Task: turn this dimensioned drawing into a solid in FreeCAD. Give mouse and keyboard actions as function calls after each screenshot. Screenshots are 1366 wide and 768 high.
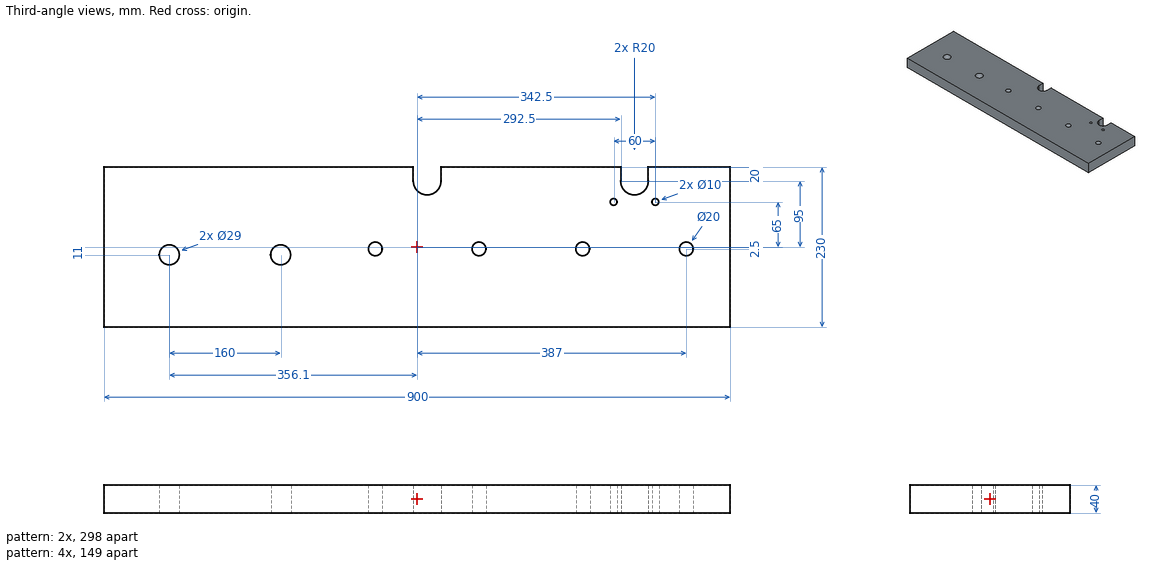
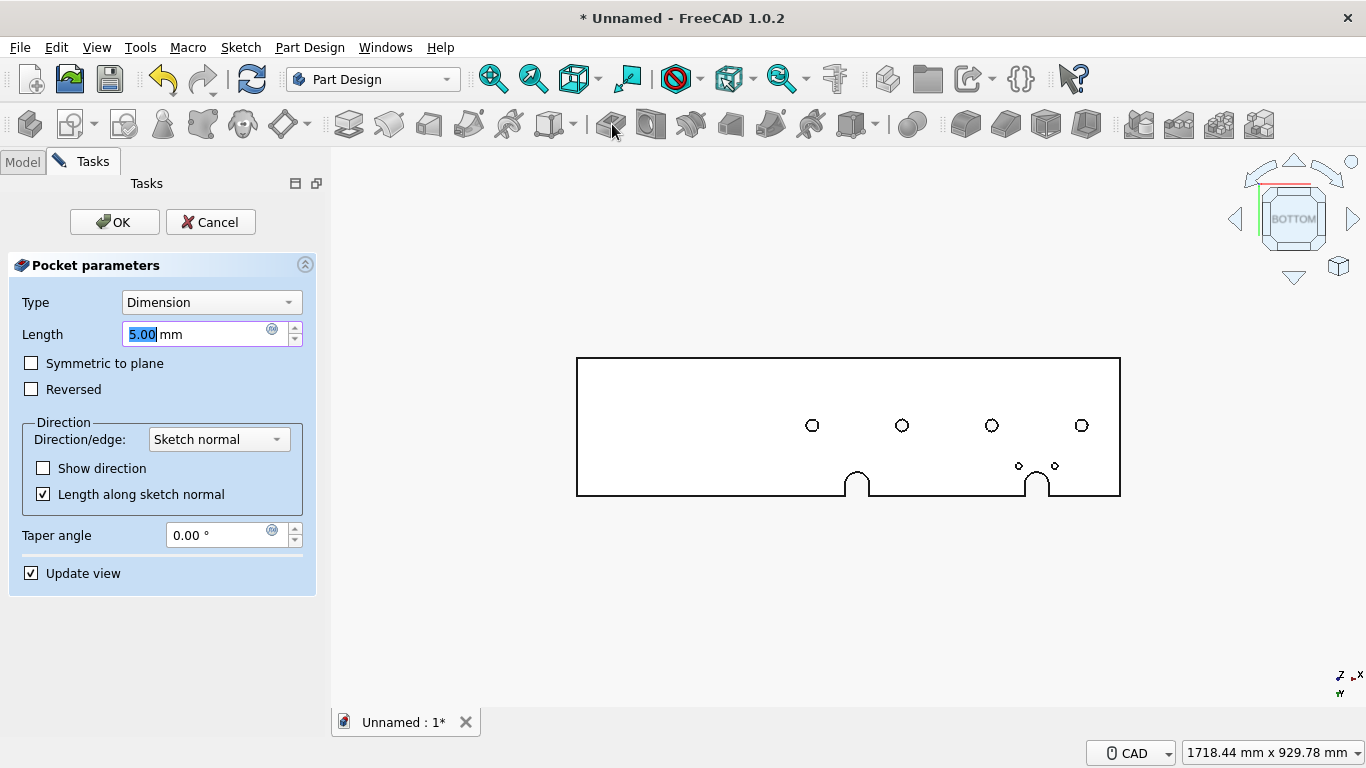
click(212, 302)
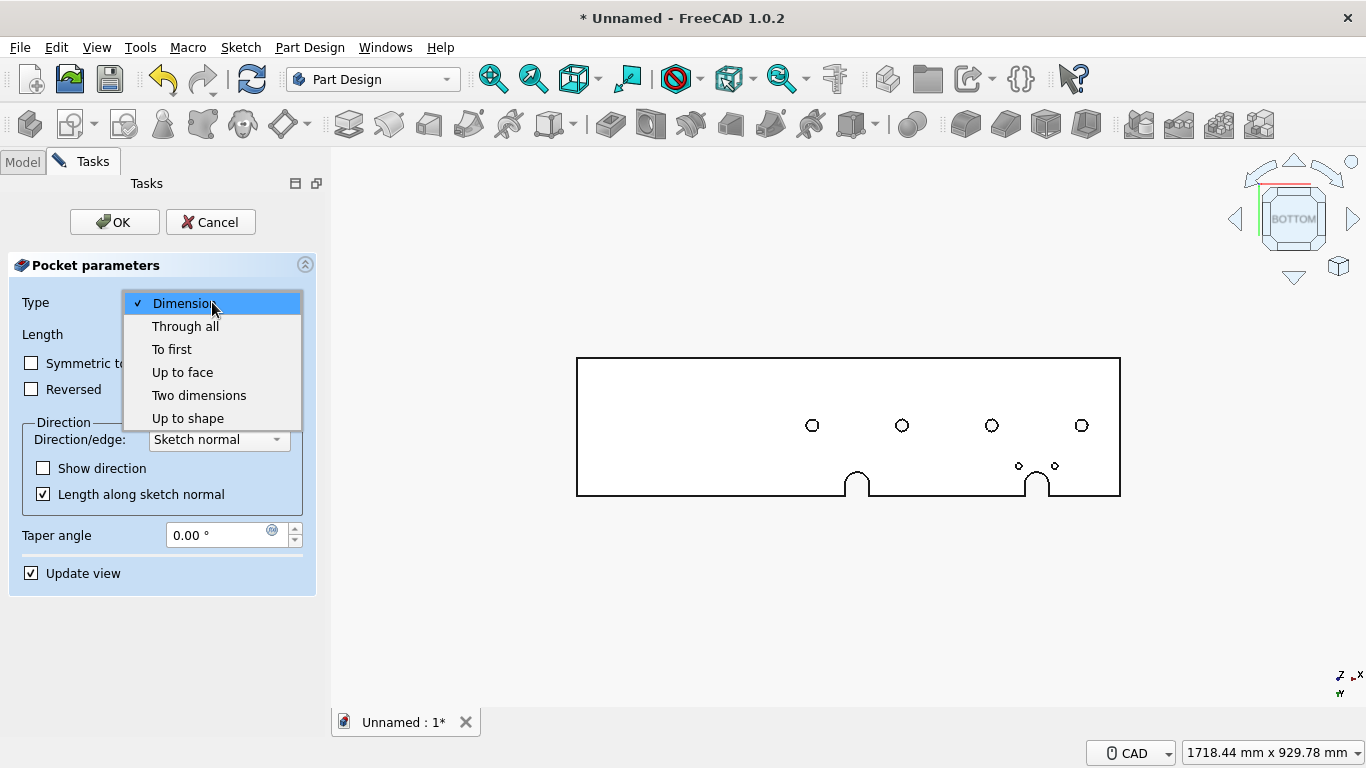
click(212, 326)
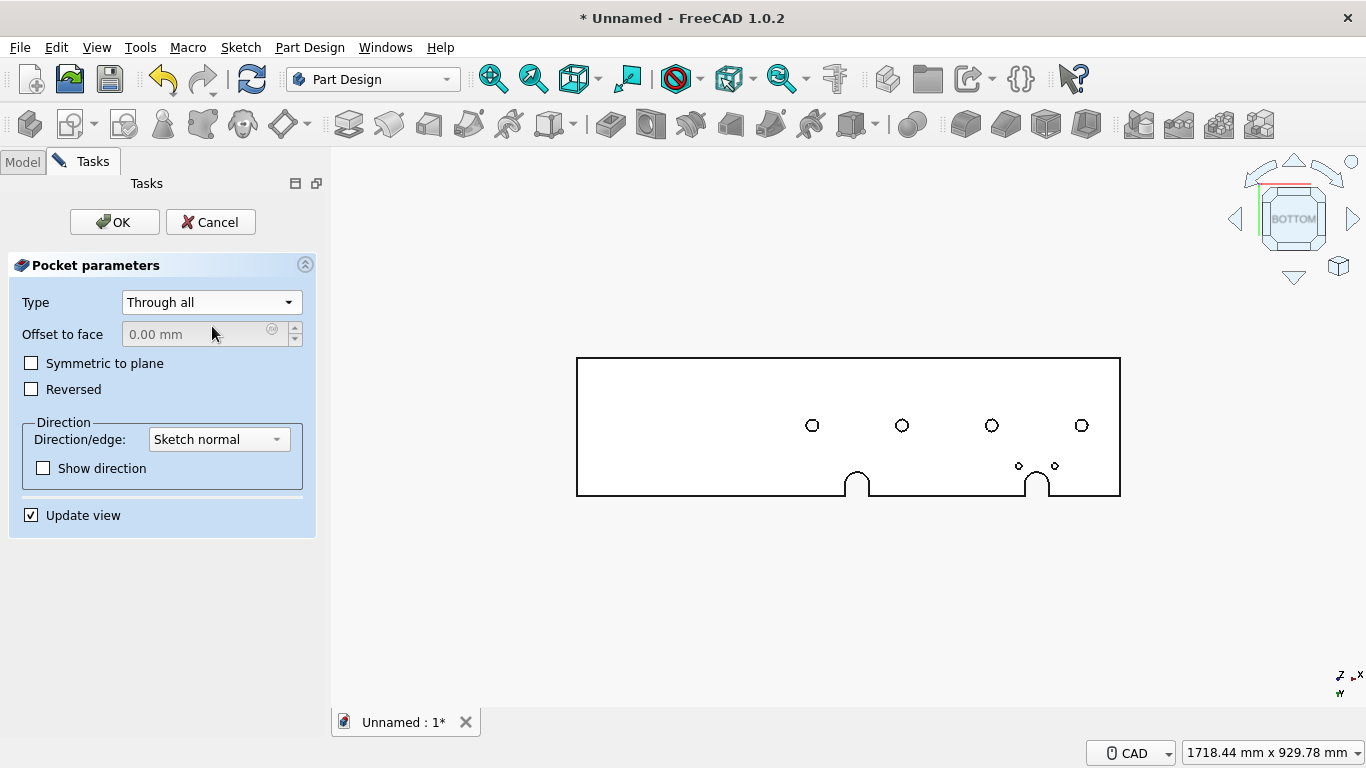
click(115, 222)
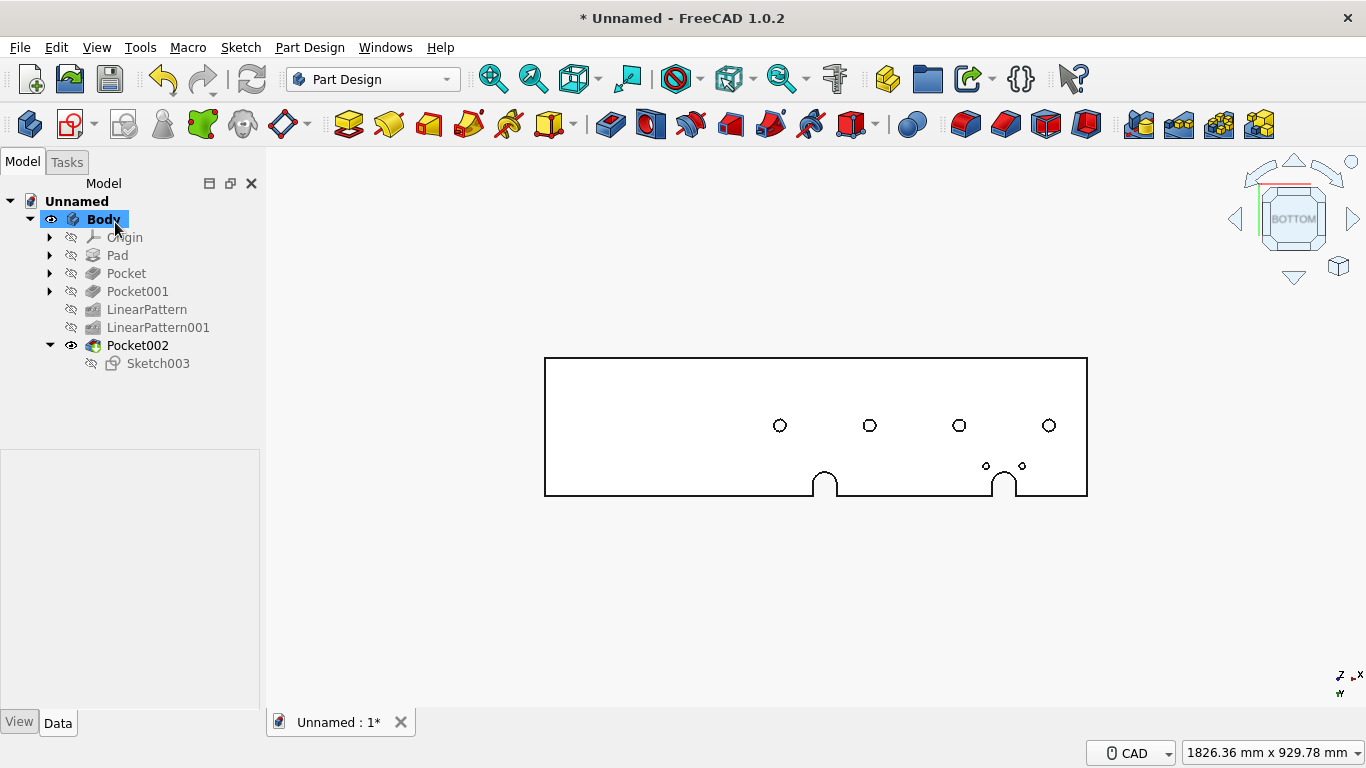
click(661, 426)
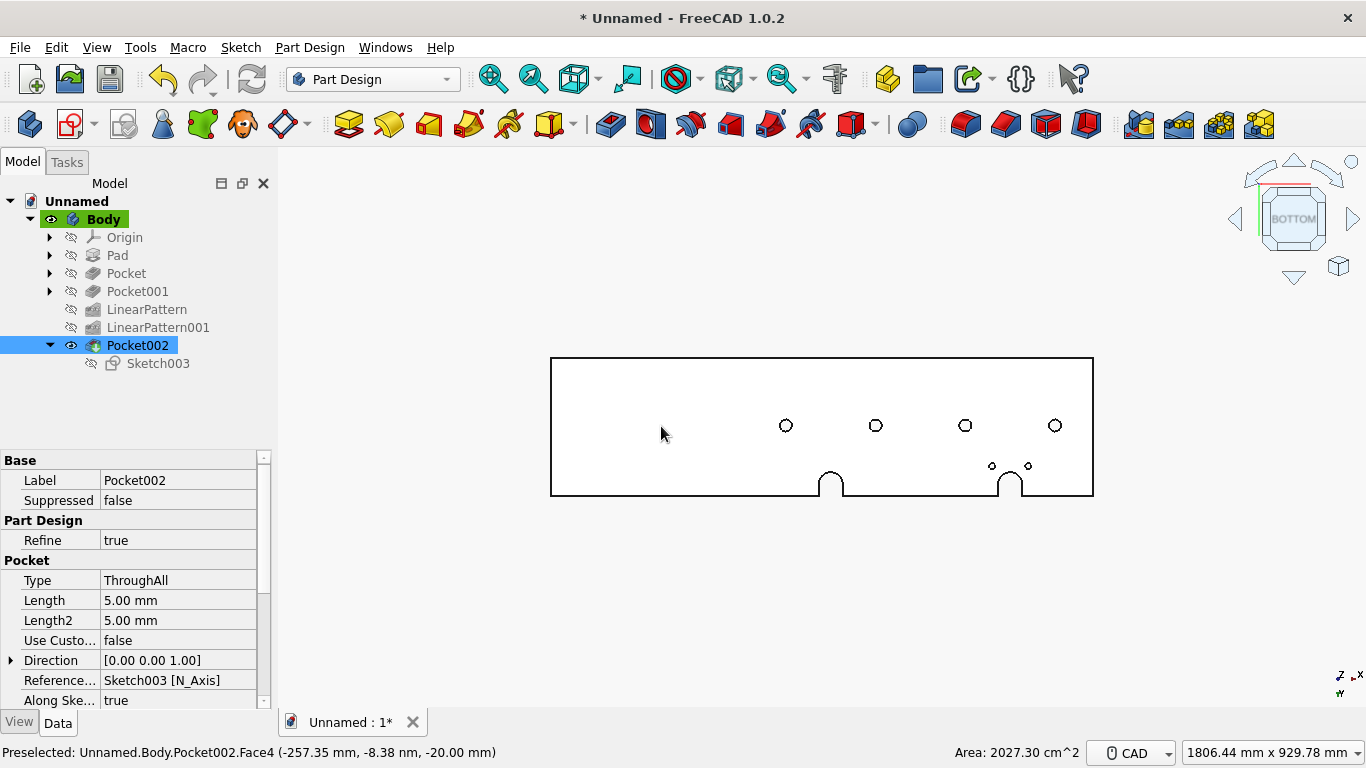
click(70, 124)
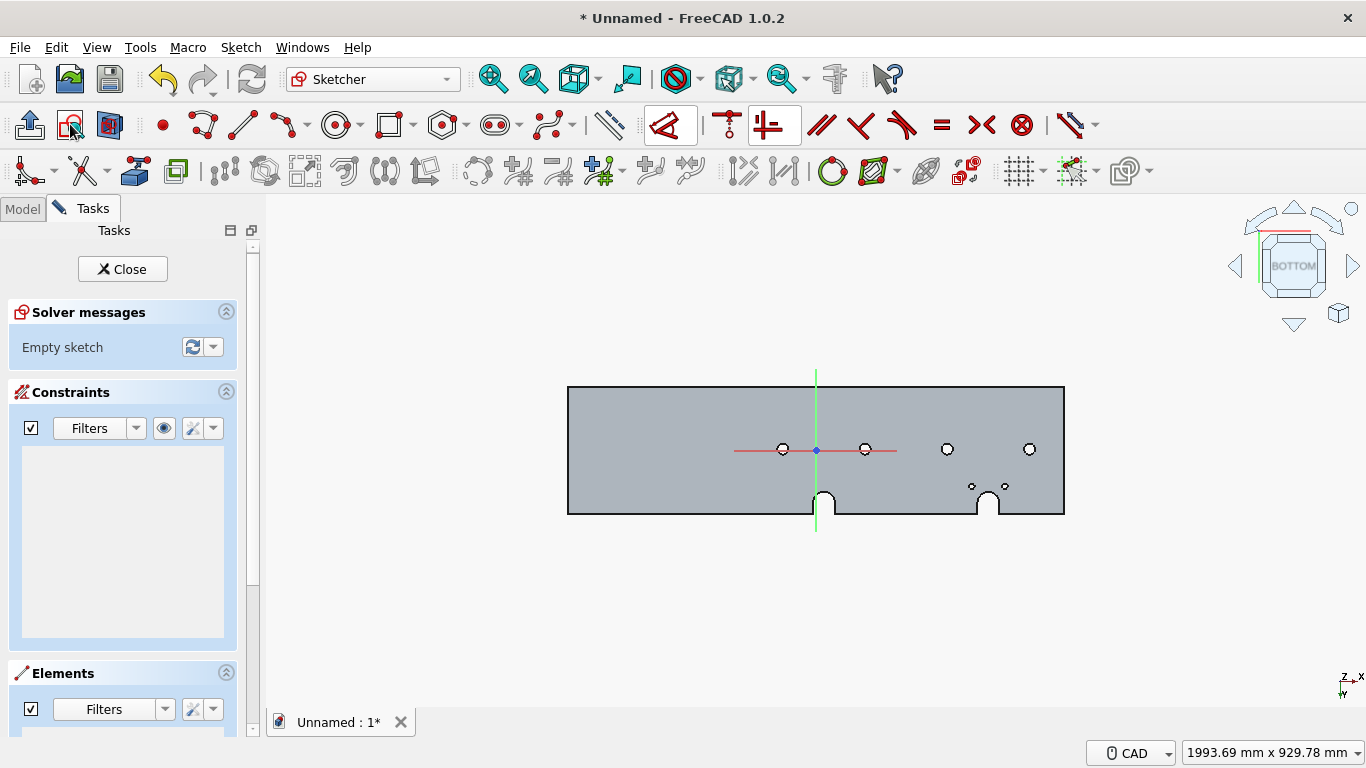
scroll(699, 442, up, 6)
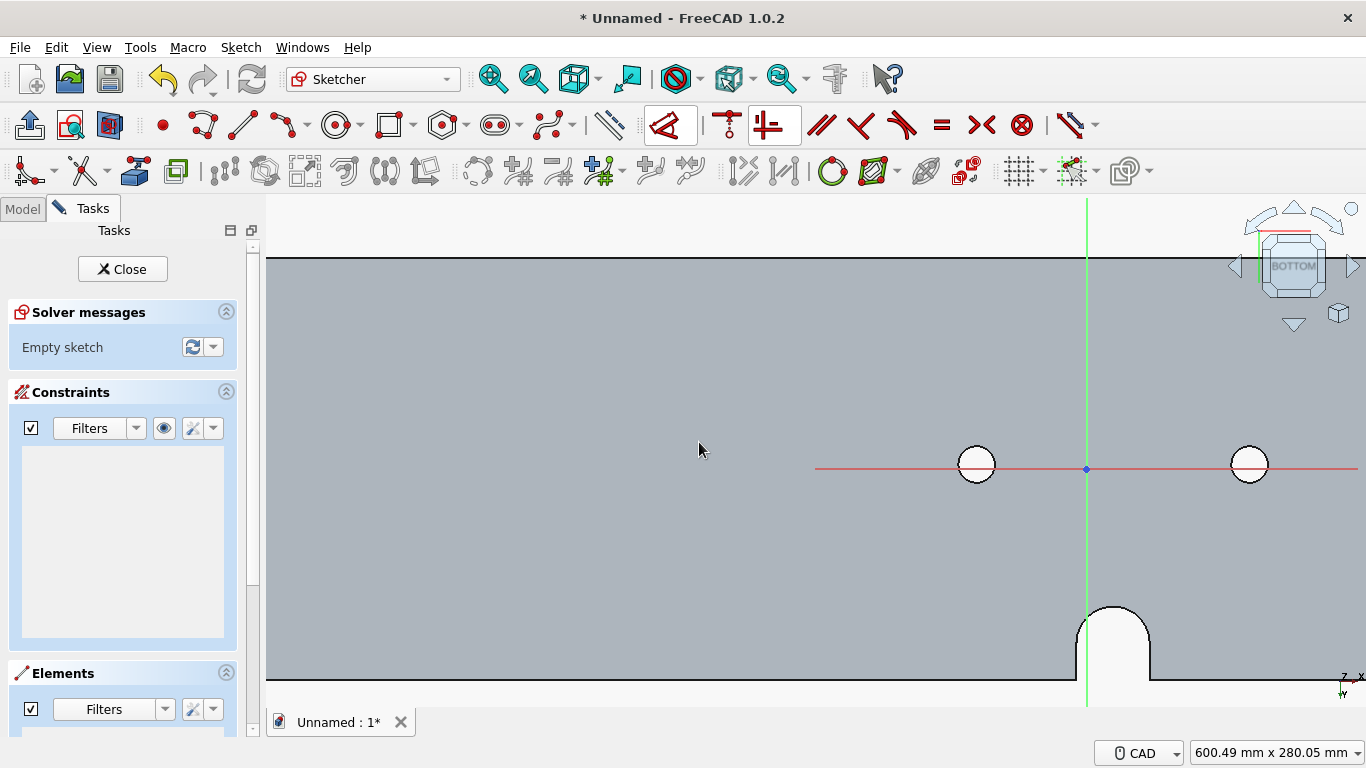
click(336, 126)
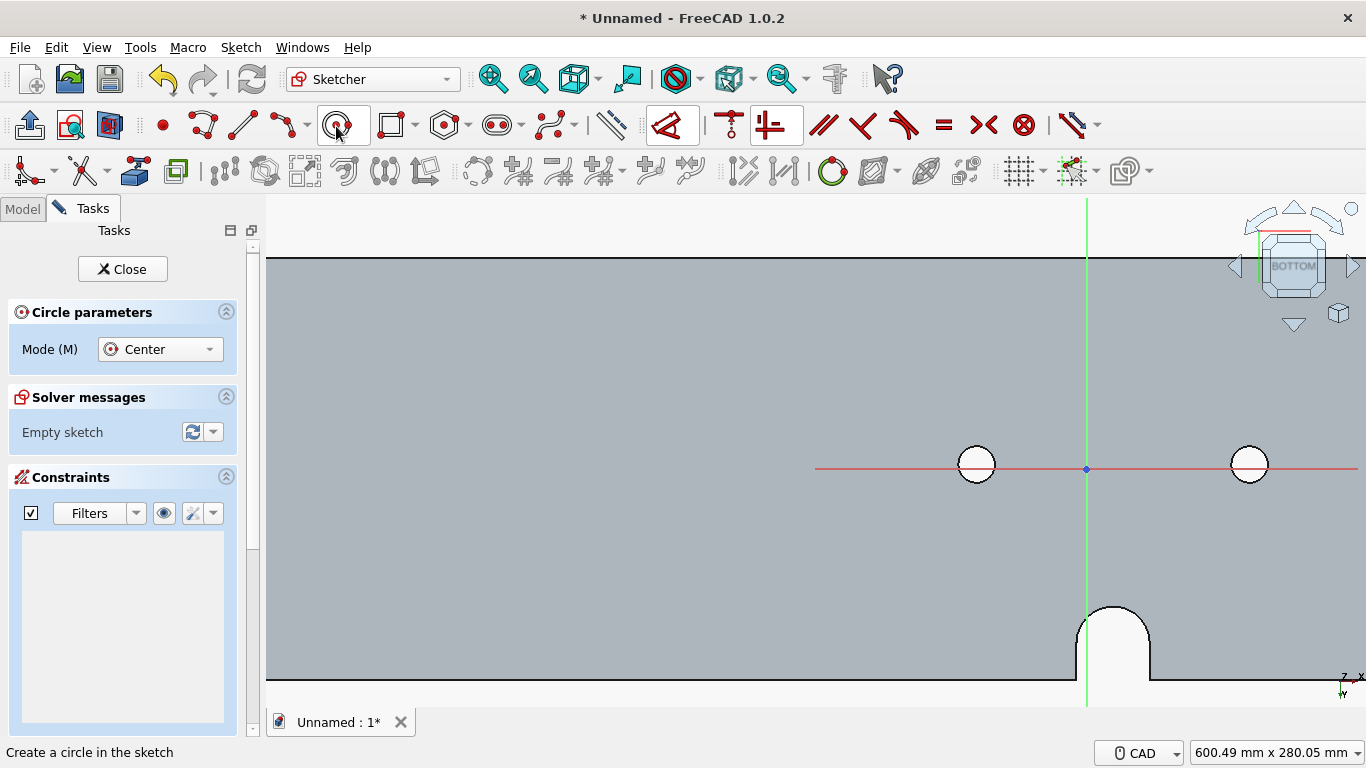
click(434, 449)
move(453, 430)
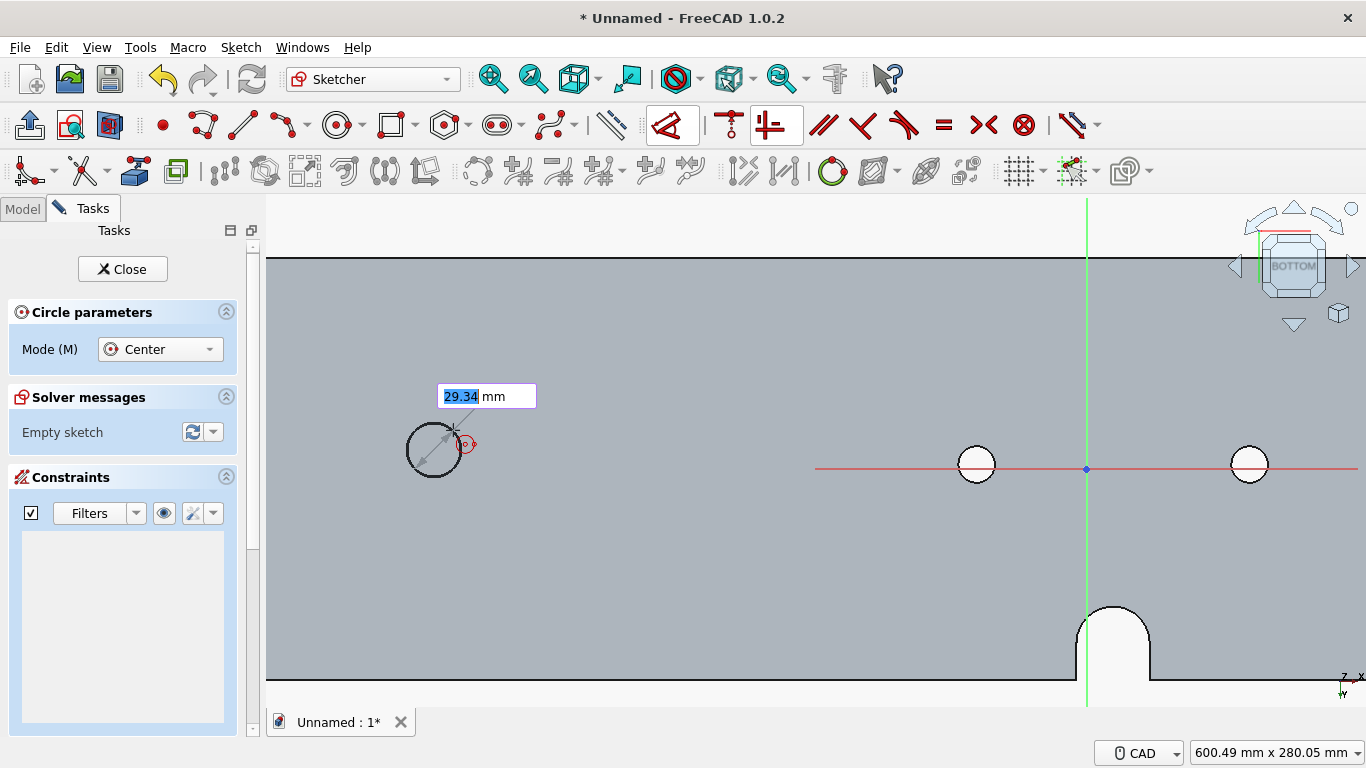
text(29)
key(Return)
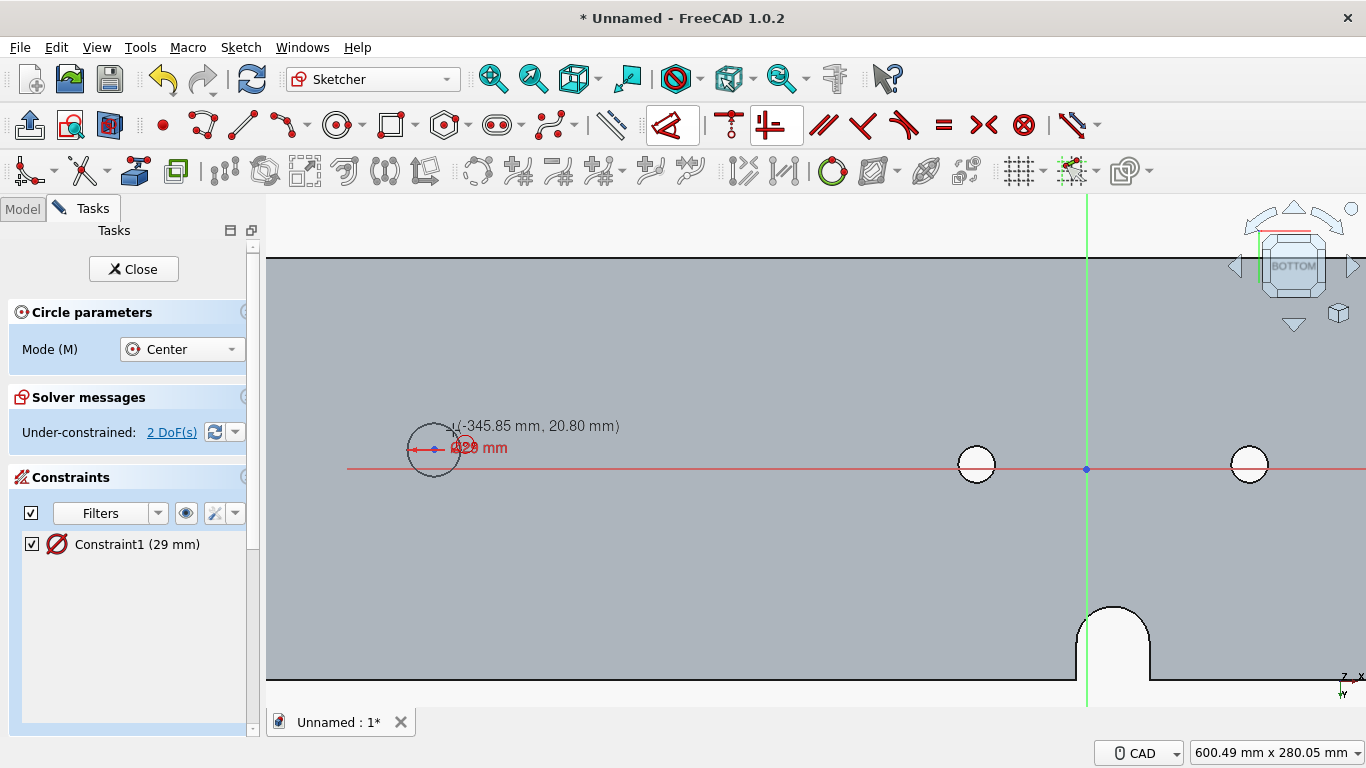
click(727, 449)
move(746, 430)